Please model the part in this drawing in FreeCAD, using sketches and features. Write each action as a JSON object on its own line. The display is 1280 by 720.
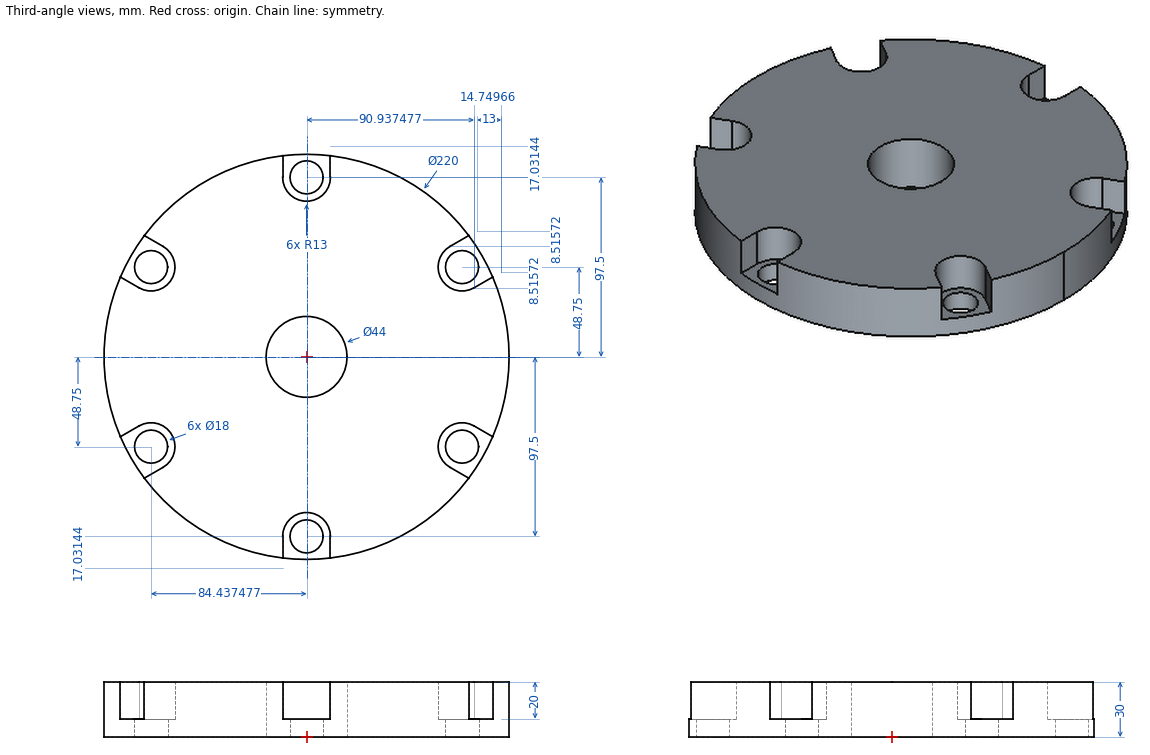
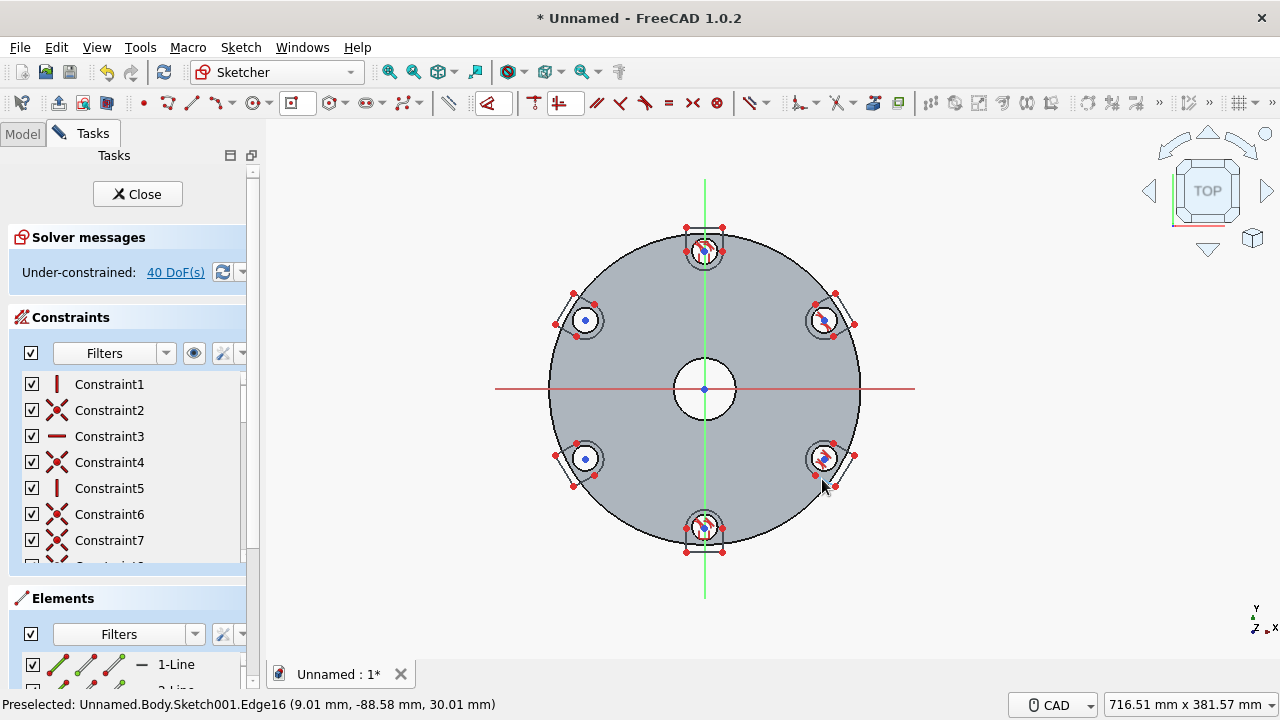
{"action": "scroll", "coordinate": [570, 447], "scroll_direction": "up", "scroll_amount": 4}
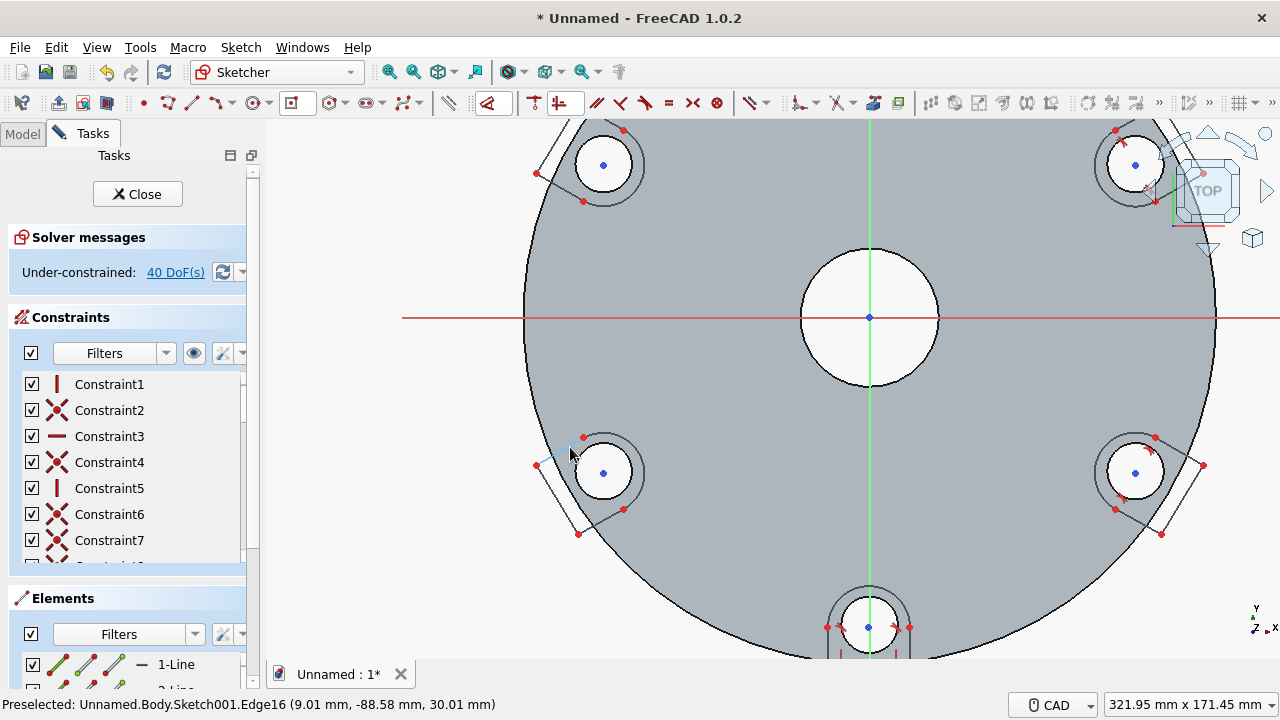
{"action": "left_click", "coordinate": [570, 446]}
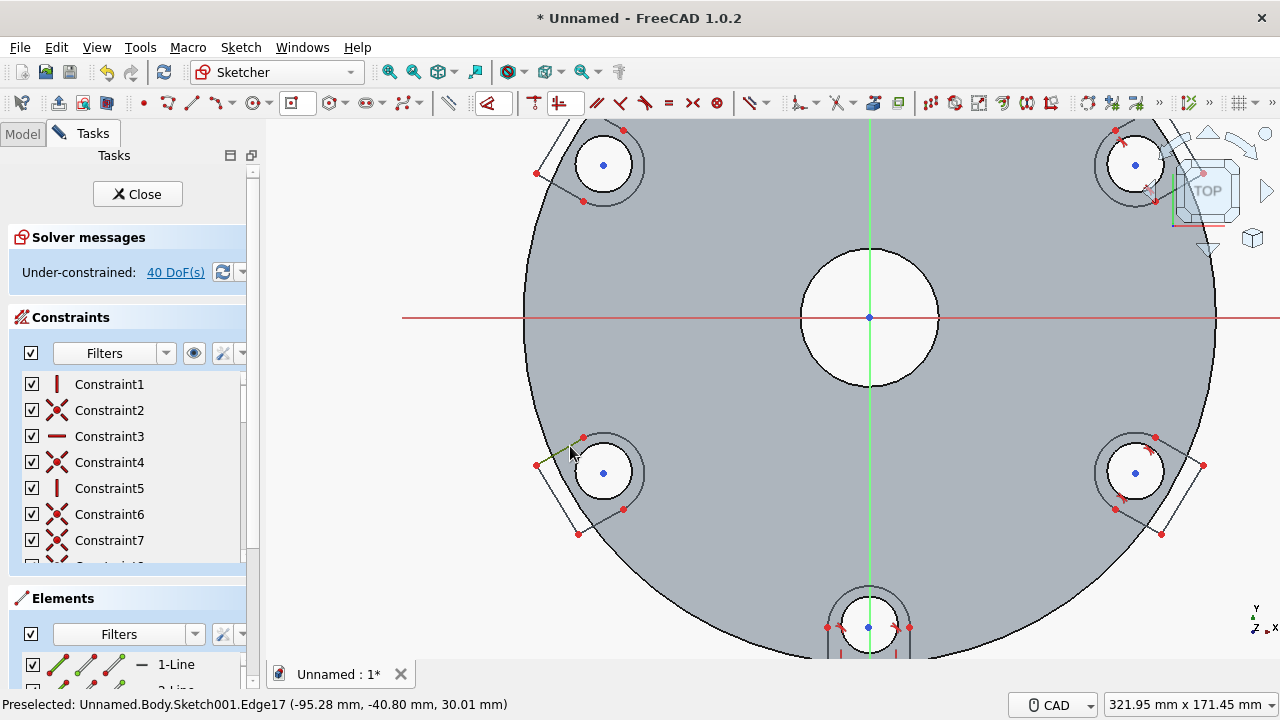
{"action": "left_click", "coordinate": [644, 478]}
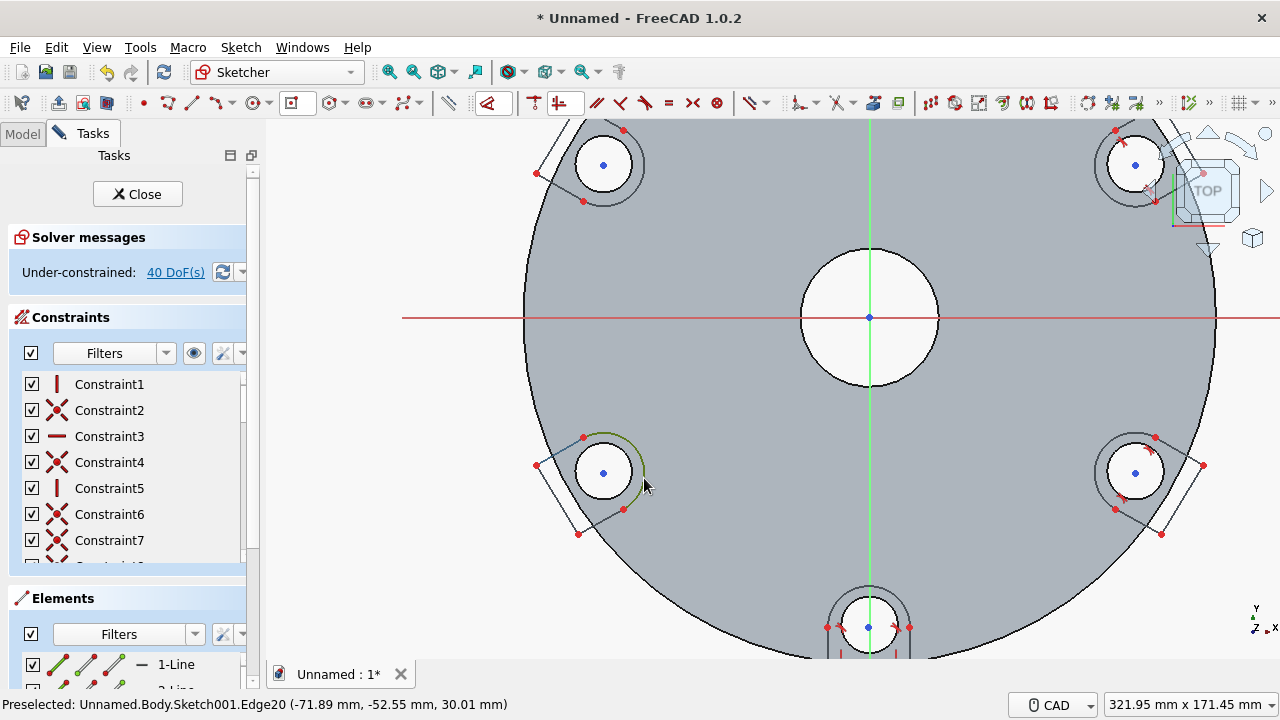
{"action": "left_click", "coordinate": [646, 104]}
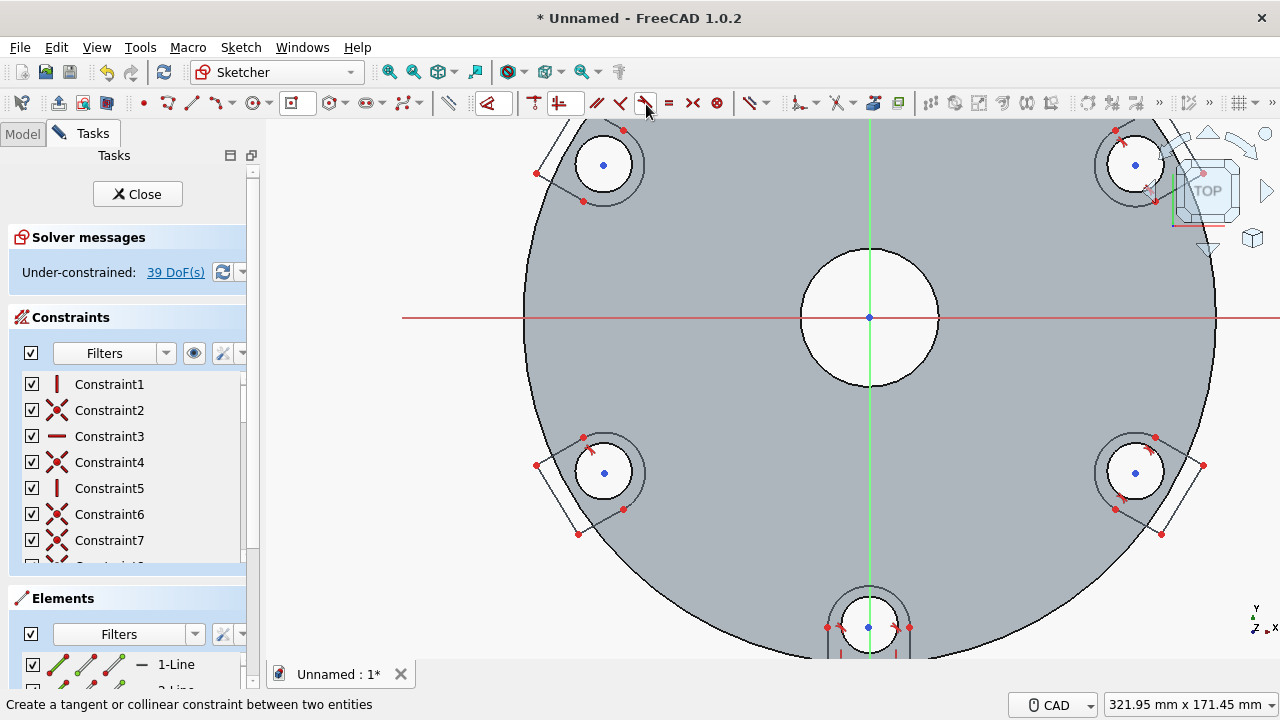
{"action": "left_click", "coordinate": [592, 527]}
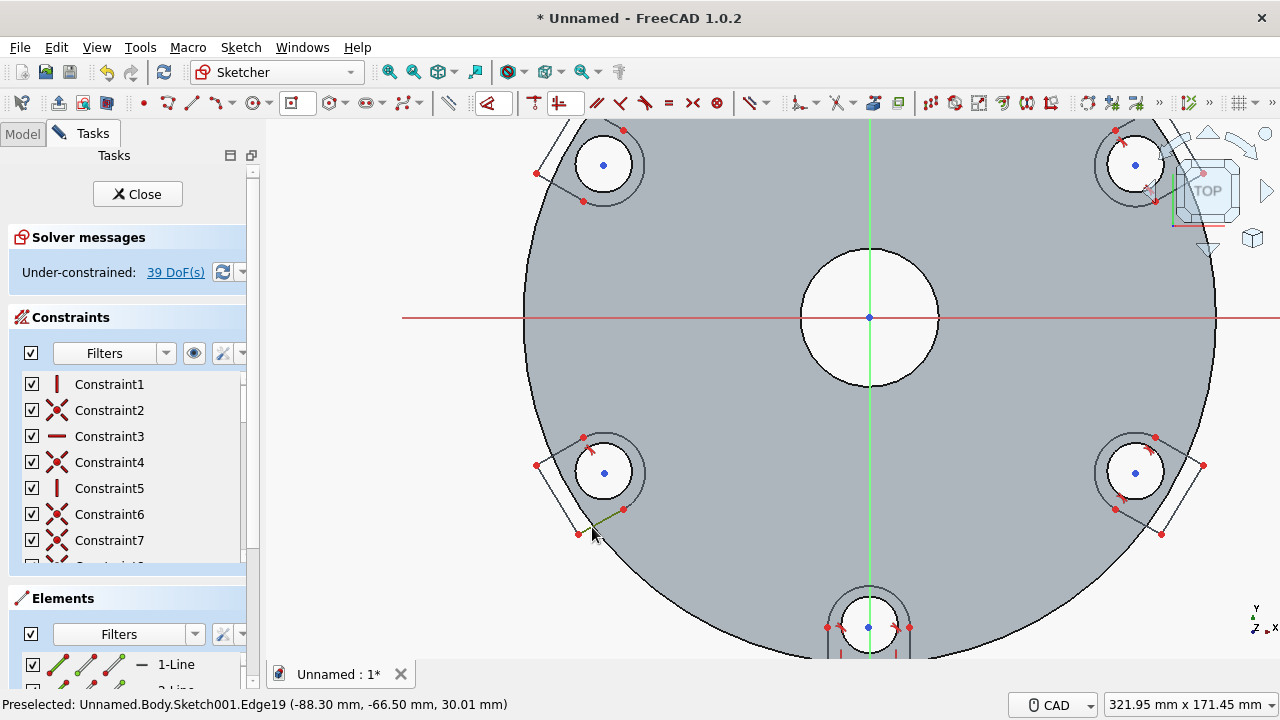
{"action": "left_click", "coordinate": [645, 478]}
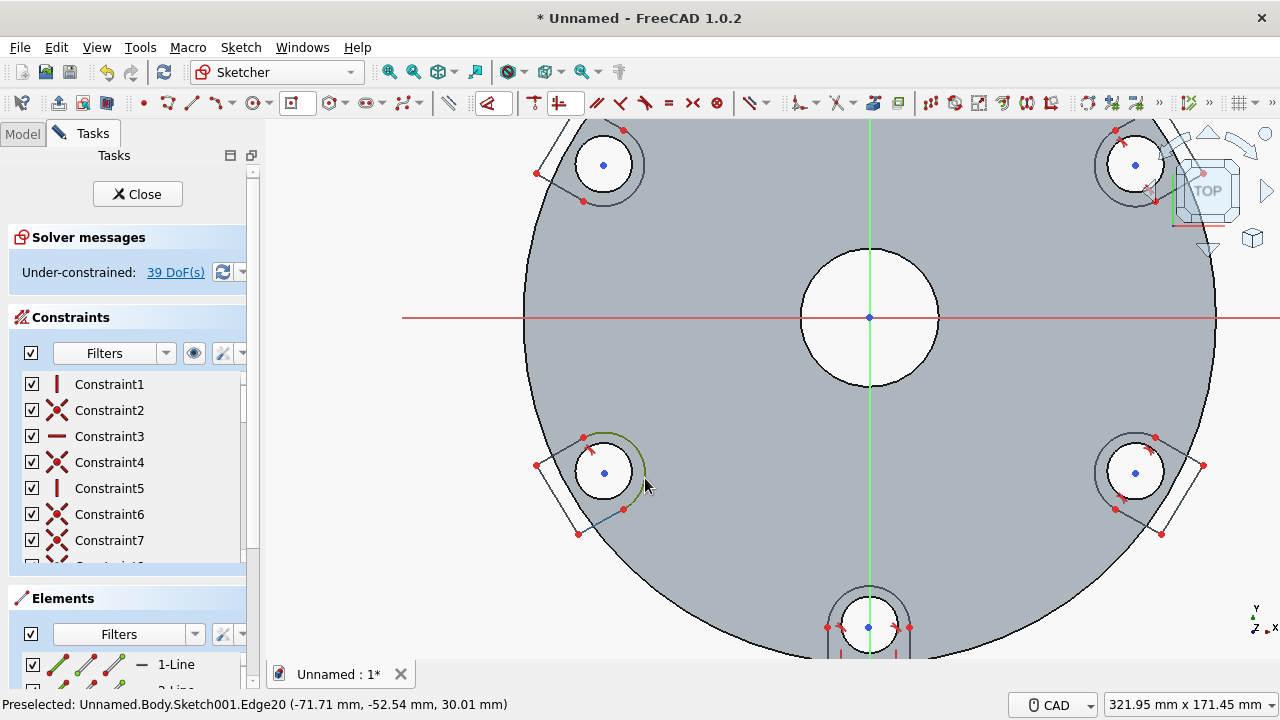
{"action": "left_click", "coordinate": [646, 104]}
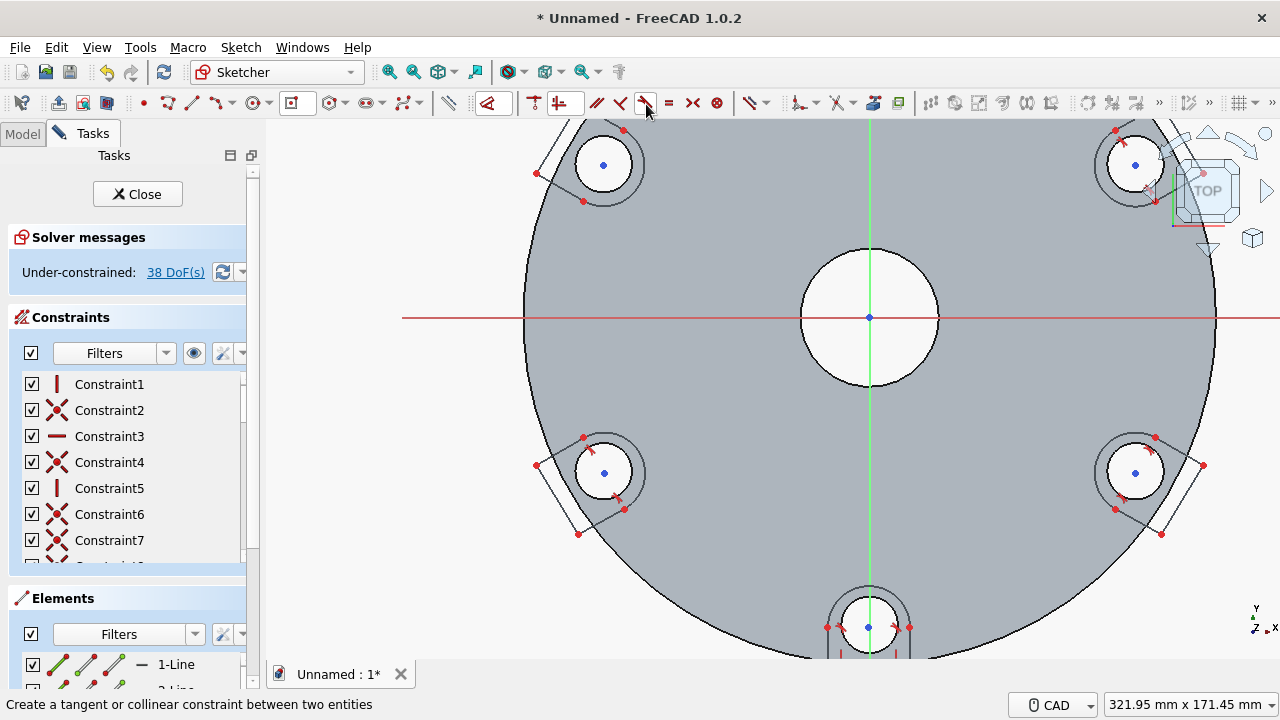
{"action": "scroll", "coordinate": [570, 447], "scroll_direction": "down", "scroll_amount": 4}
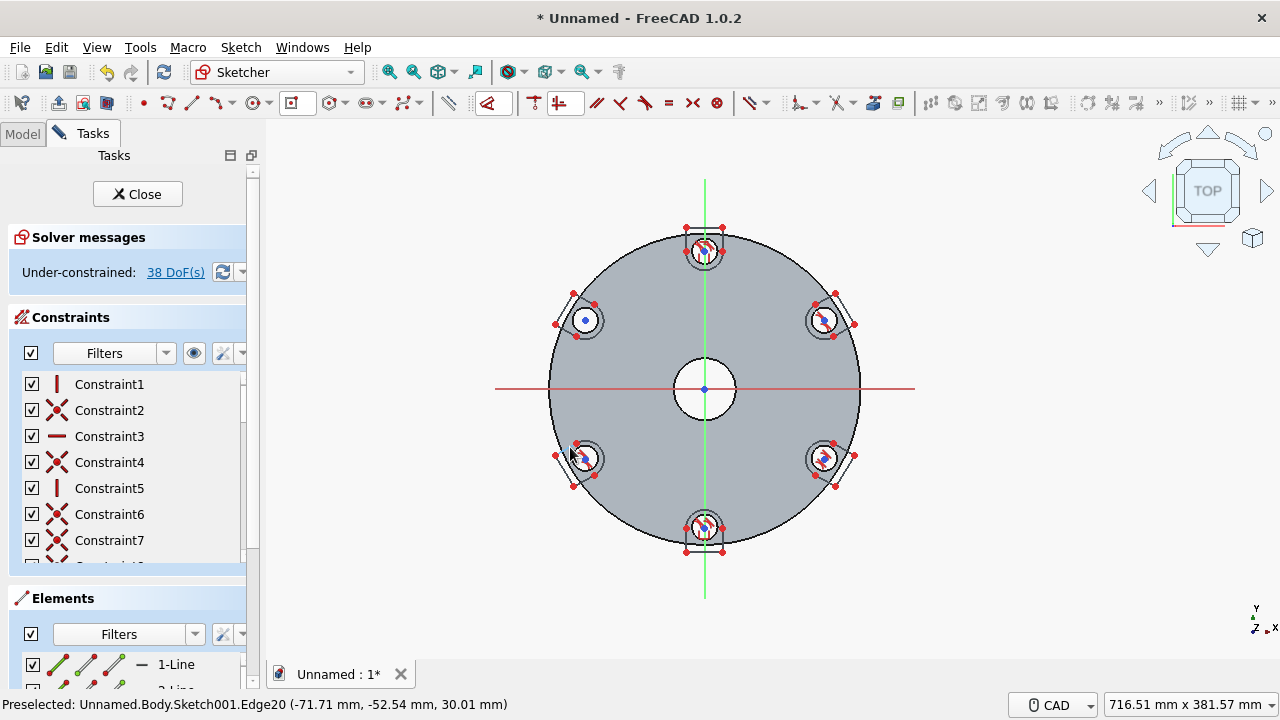
{"action": "scroll", "coordinate": [588, 301], "scroll_direction": "up", "scroll_amount": 4}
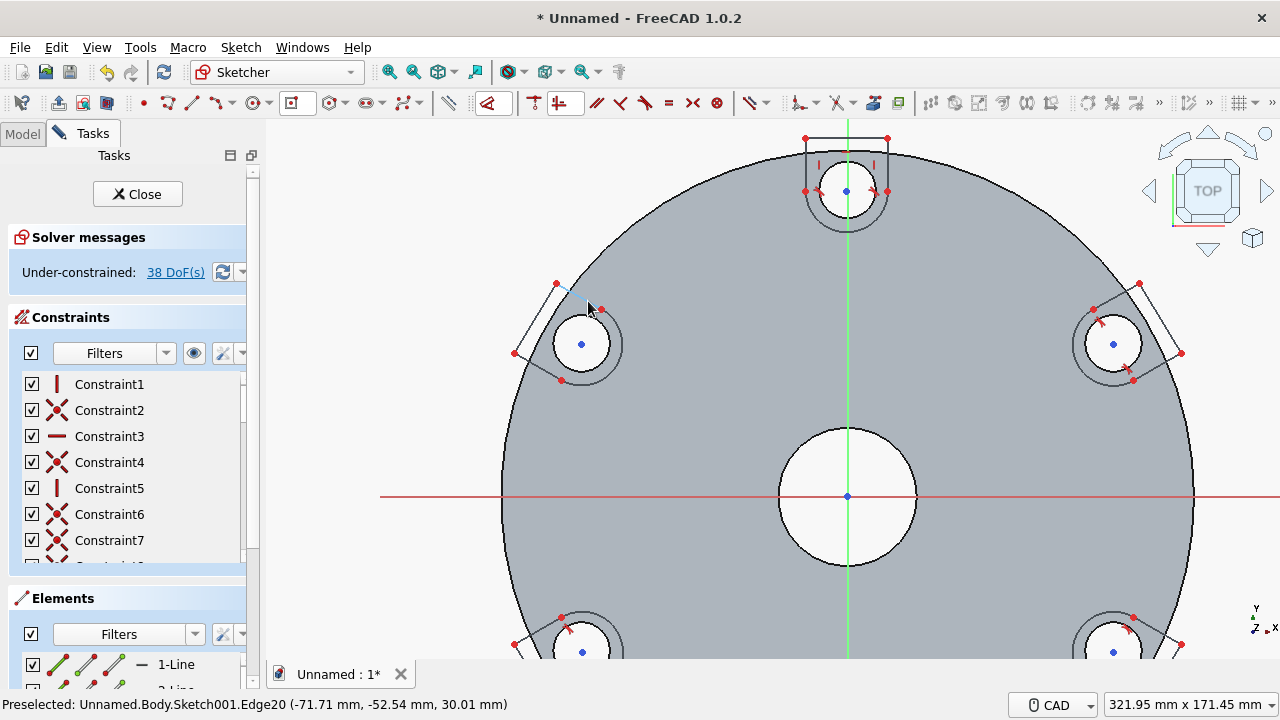
{"action": "left_click", "coordinate": [588, 302]}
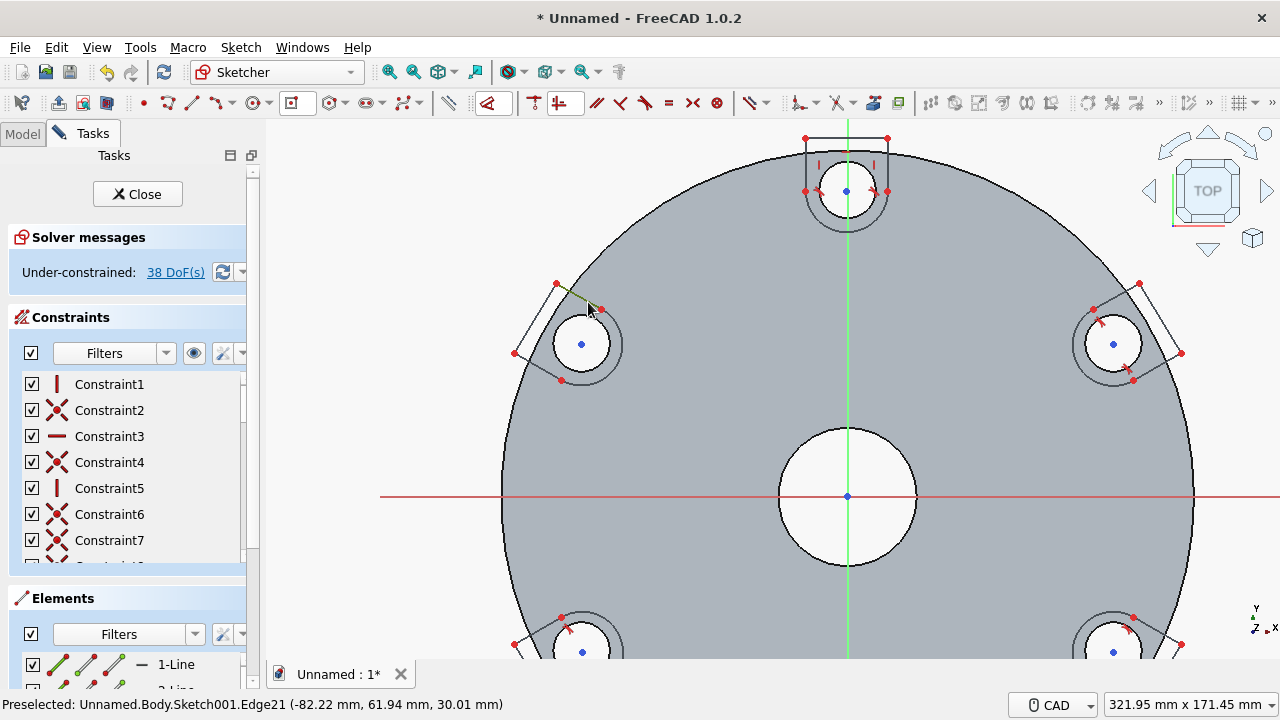
{"action": "left_click", "coordinate": [599, 382]}